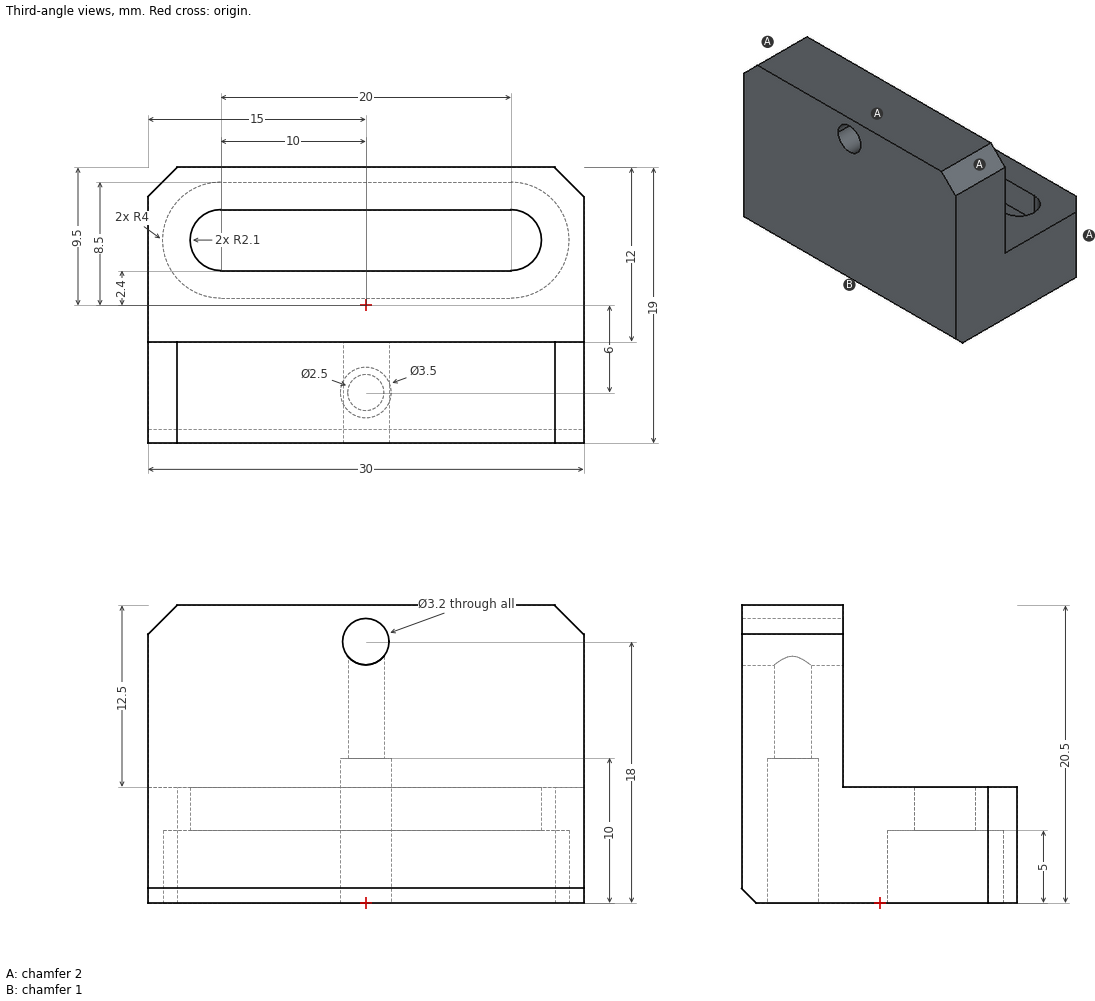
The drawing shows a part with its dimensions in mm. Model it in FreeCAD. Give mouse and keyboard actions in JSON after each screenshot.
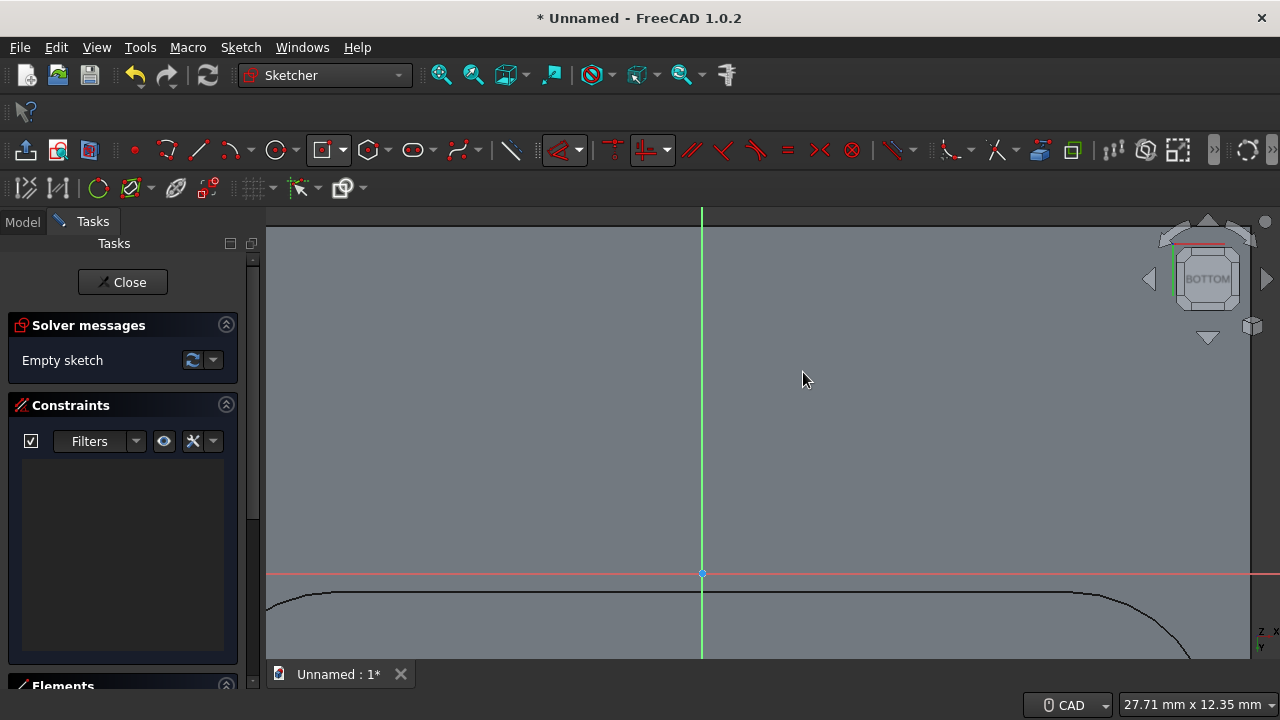
{"action": "left_click", "coordinate": [276, 150]}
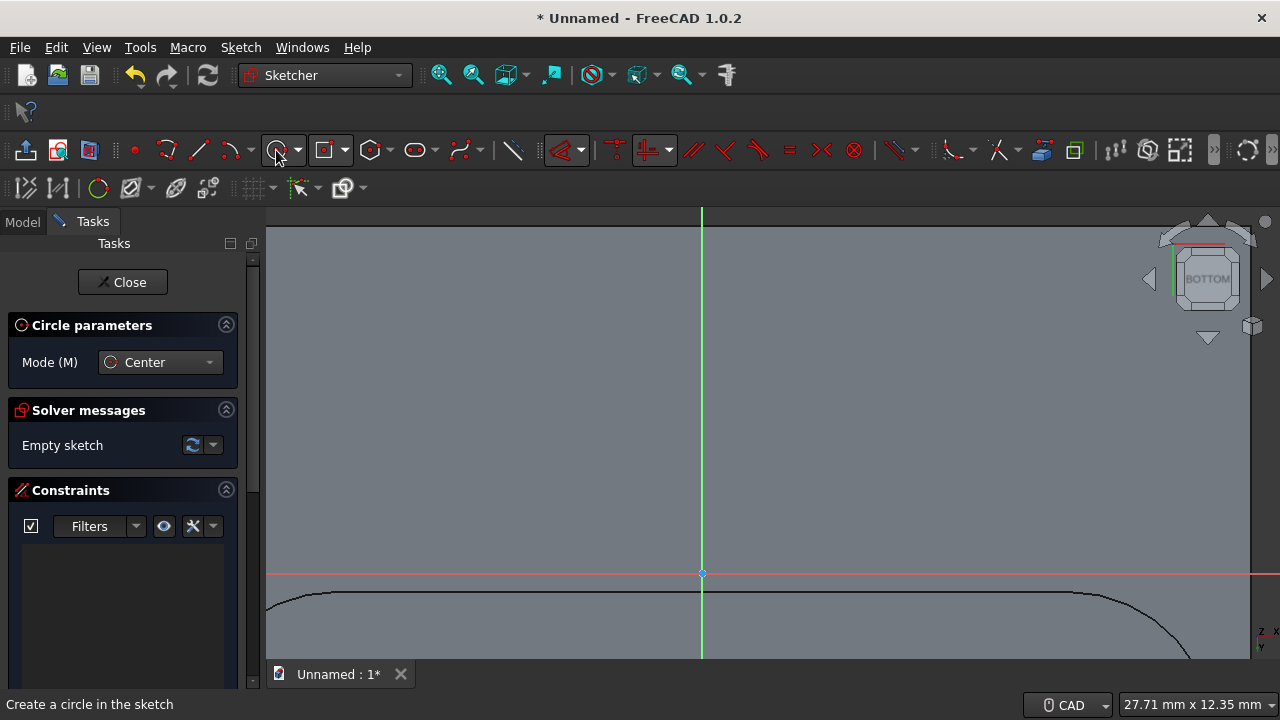
{"action": "left_click", "coordinate": [702, 354]}
{"action": "mouse_move", "coordinate": [747, 309]}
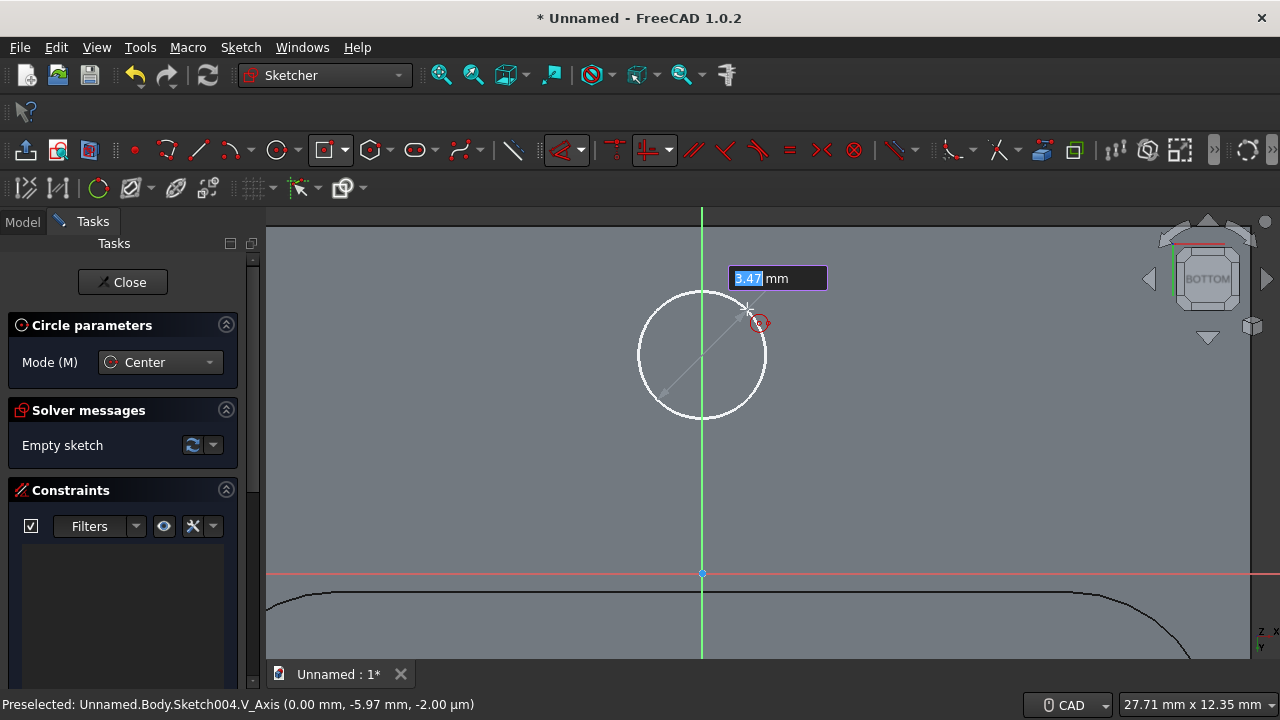
{"action": "type", "text": "3.5"}
{"action": "key", "text": "Return"}
{"action": "key", "text": "Escape"}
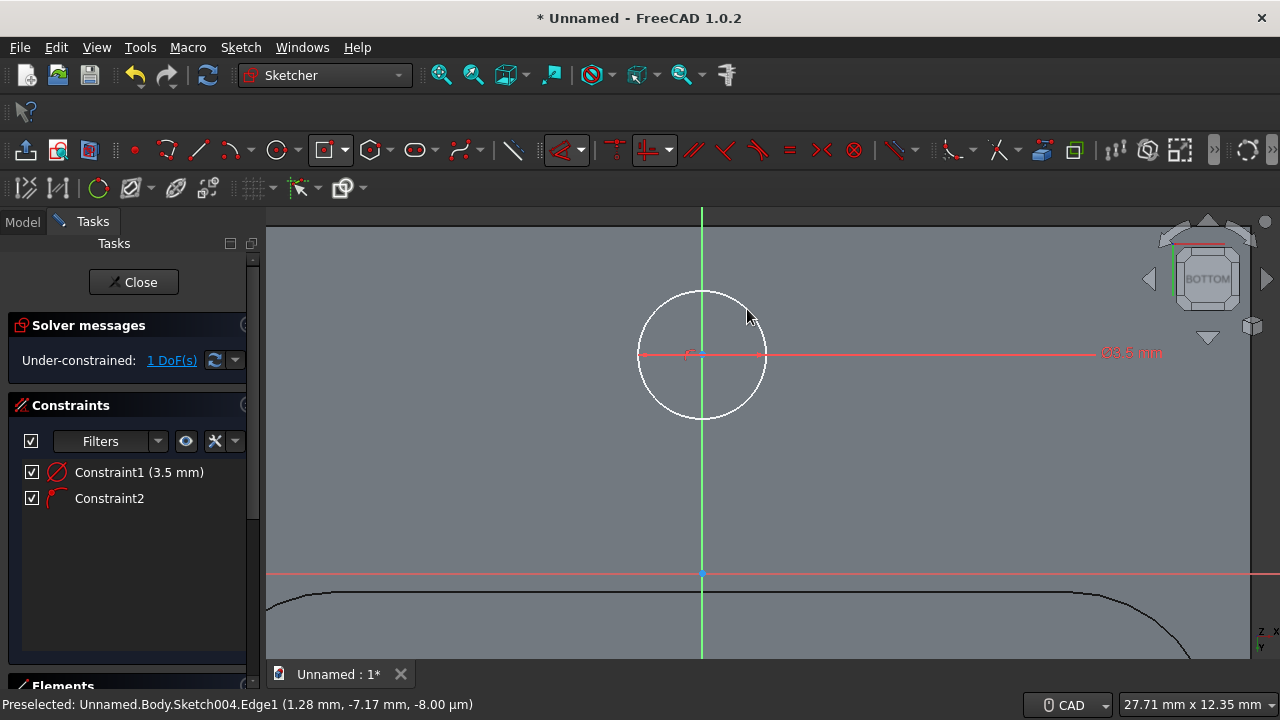
{"action": "left_click", "coordinate": [702, 355]}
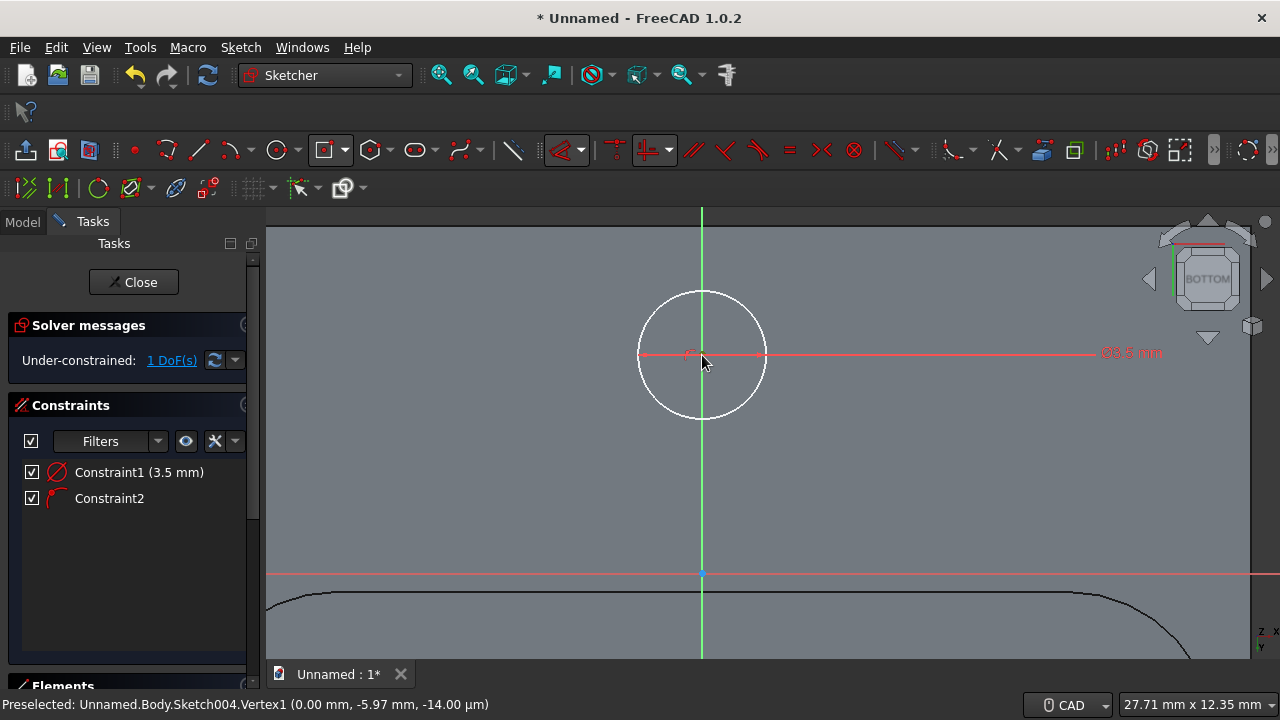
{"action": "key", "text": "i"}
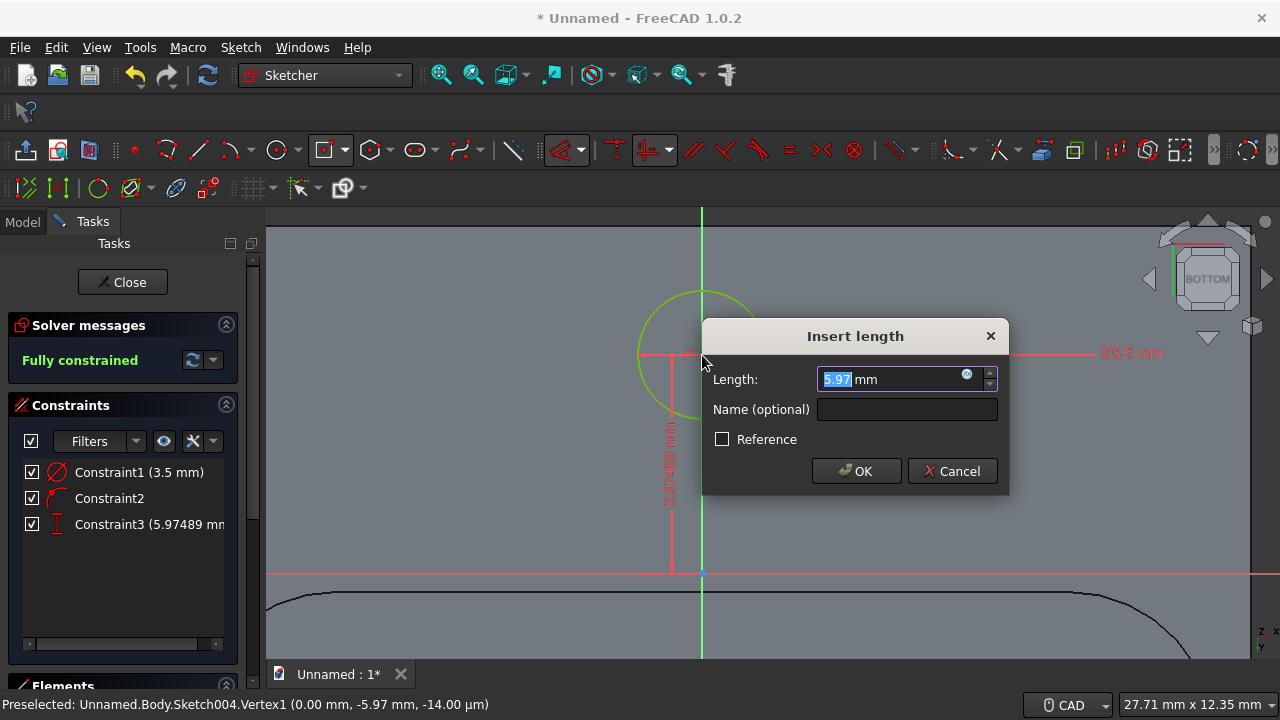
{"action": "type", "text": "6"}
{"action": "key", "text": "Return"}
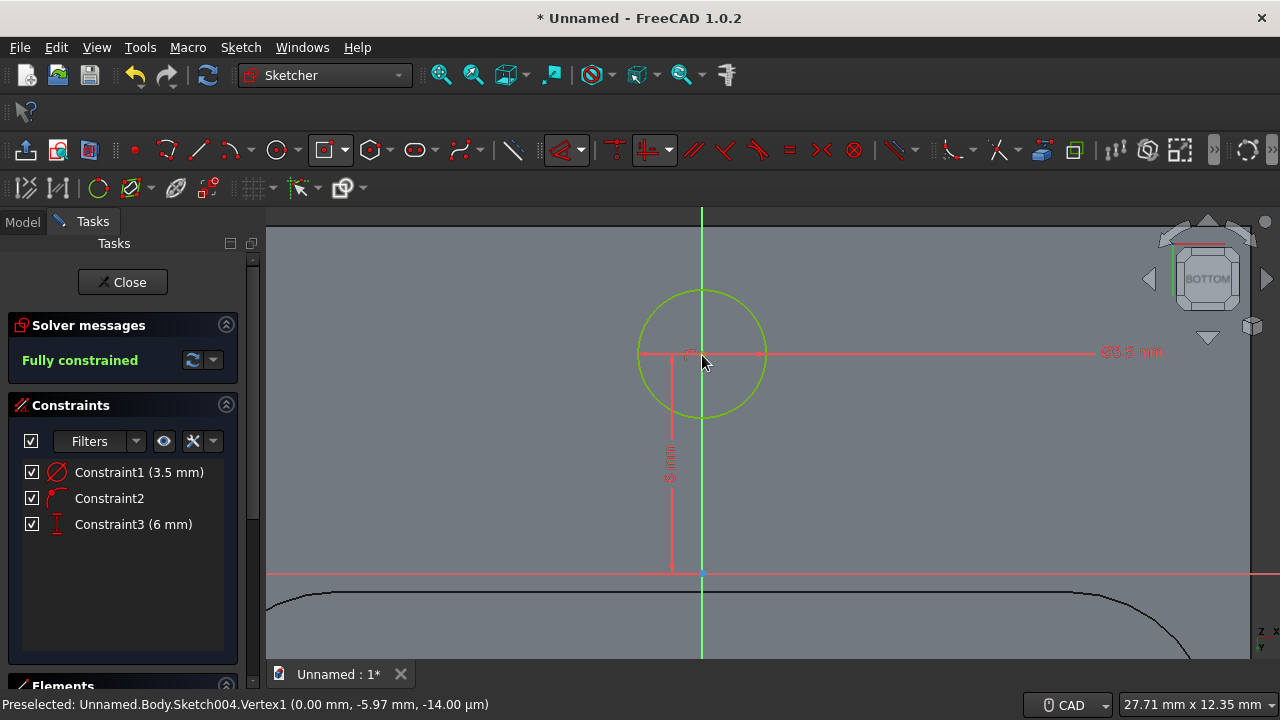
{"action": "left_click", "coordinate": [123, 282]}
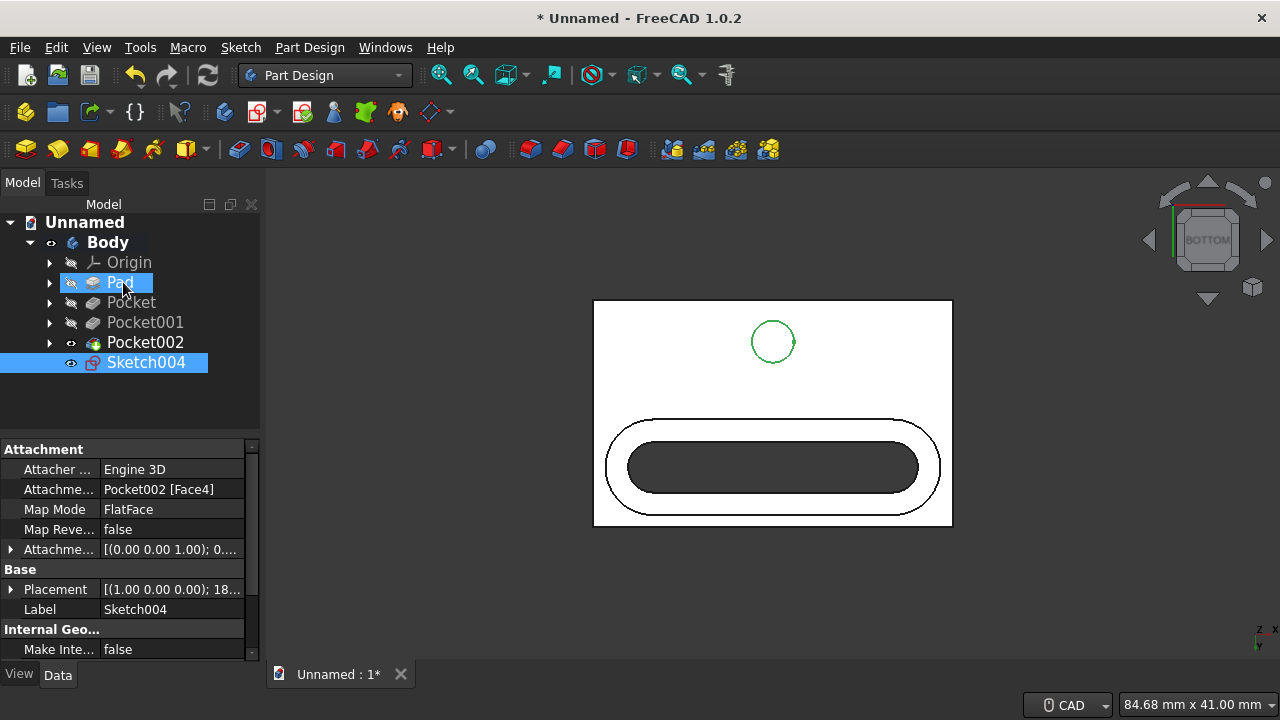
{"action": "left_click", "coordinate": [240, 150]}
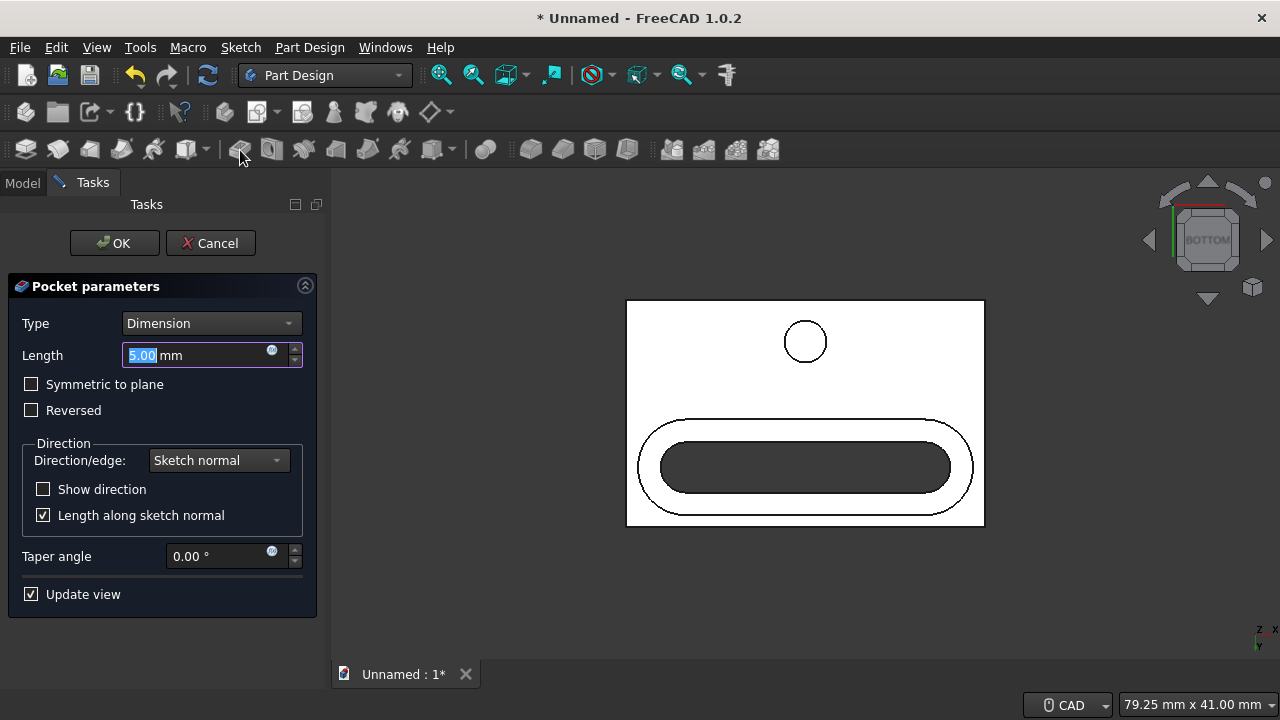
{"action": "type", "text": "10"}
{"action": "key", "text": "Tab"}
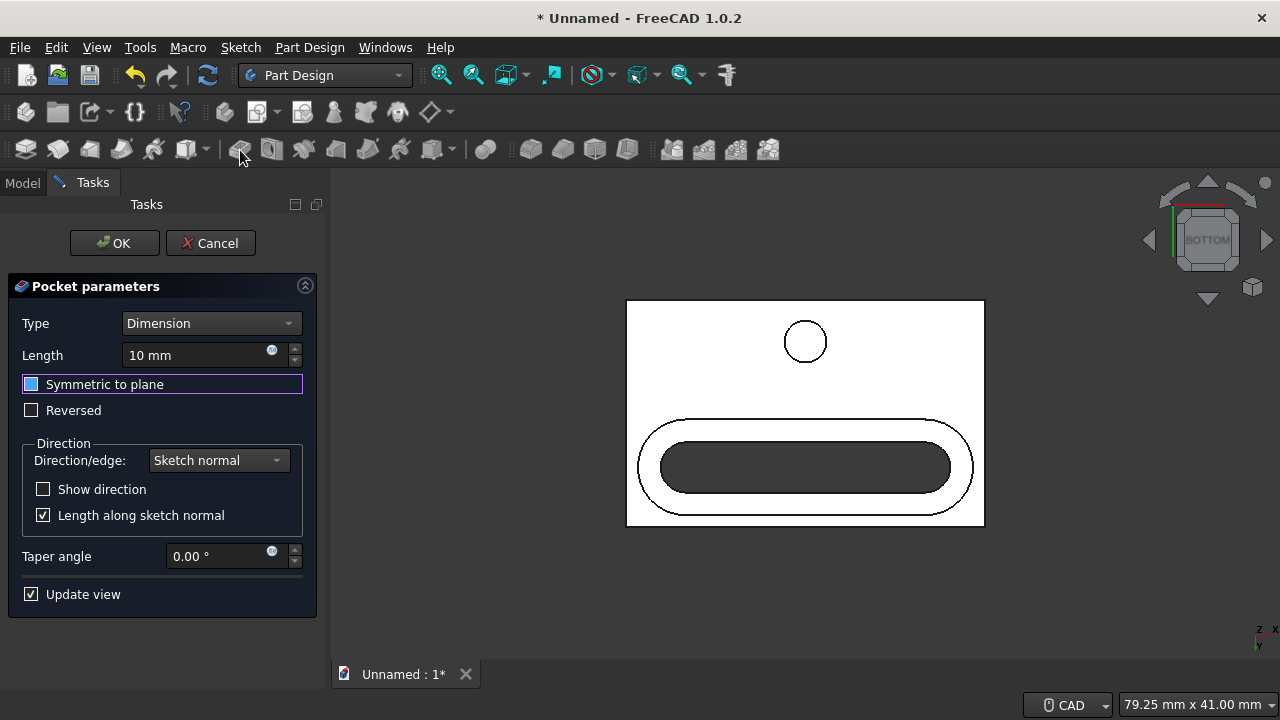
{"action": "left_click", "coordinate": [115, 243]}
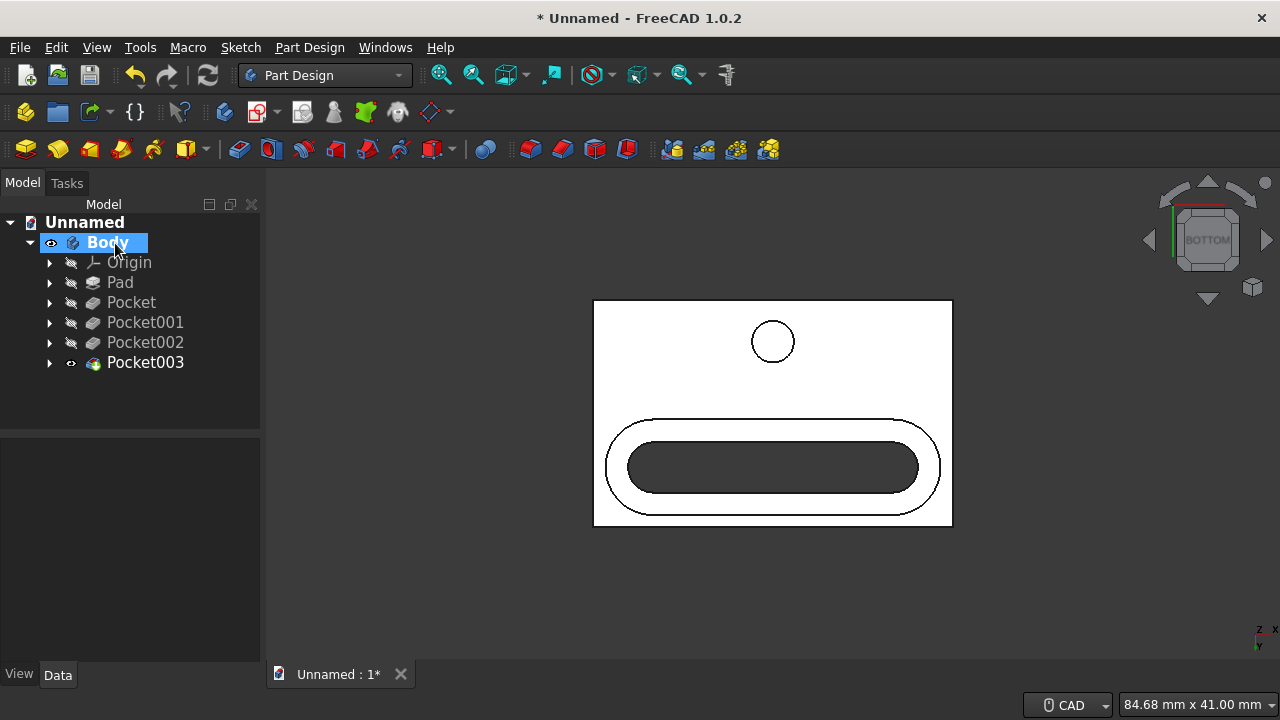
{"action": "key", "text": "0"}